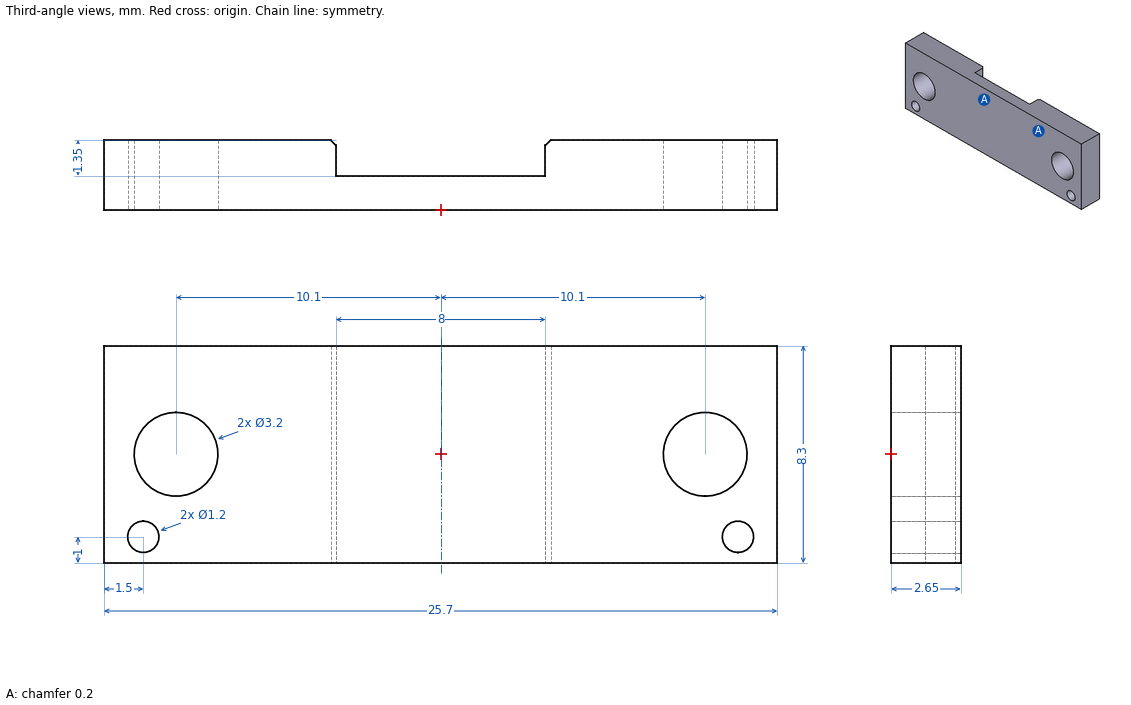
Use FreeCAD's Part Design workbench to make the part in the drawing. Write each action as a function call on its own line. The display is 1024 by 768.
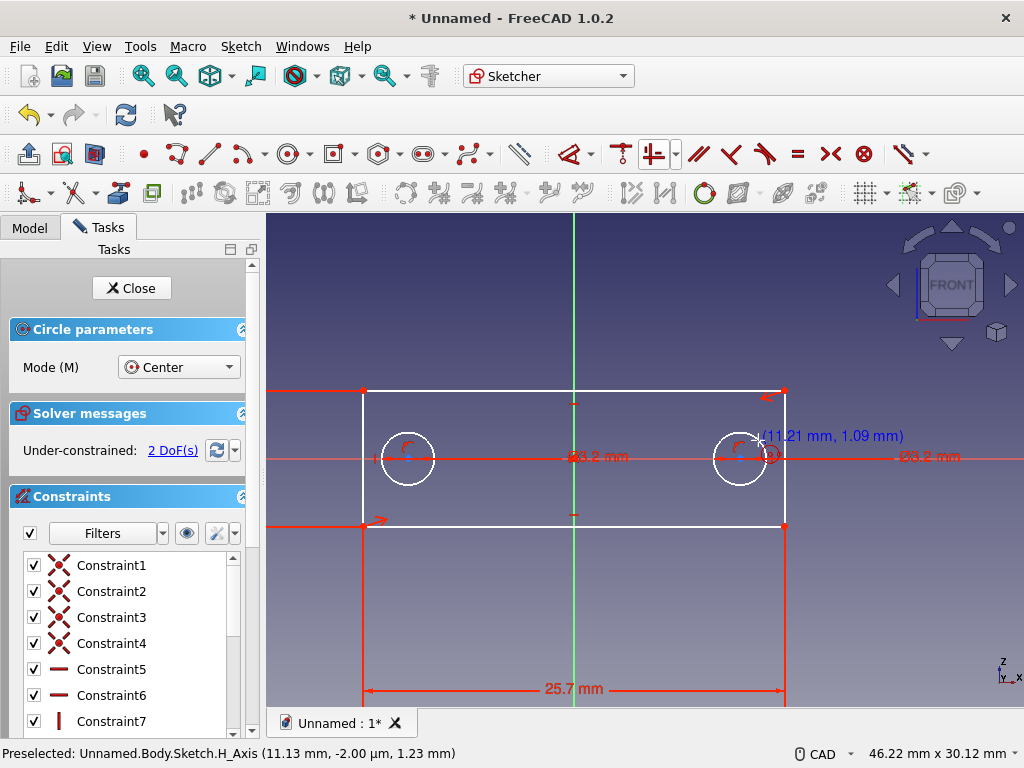
scroll(388, 511, up, 5)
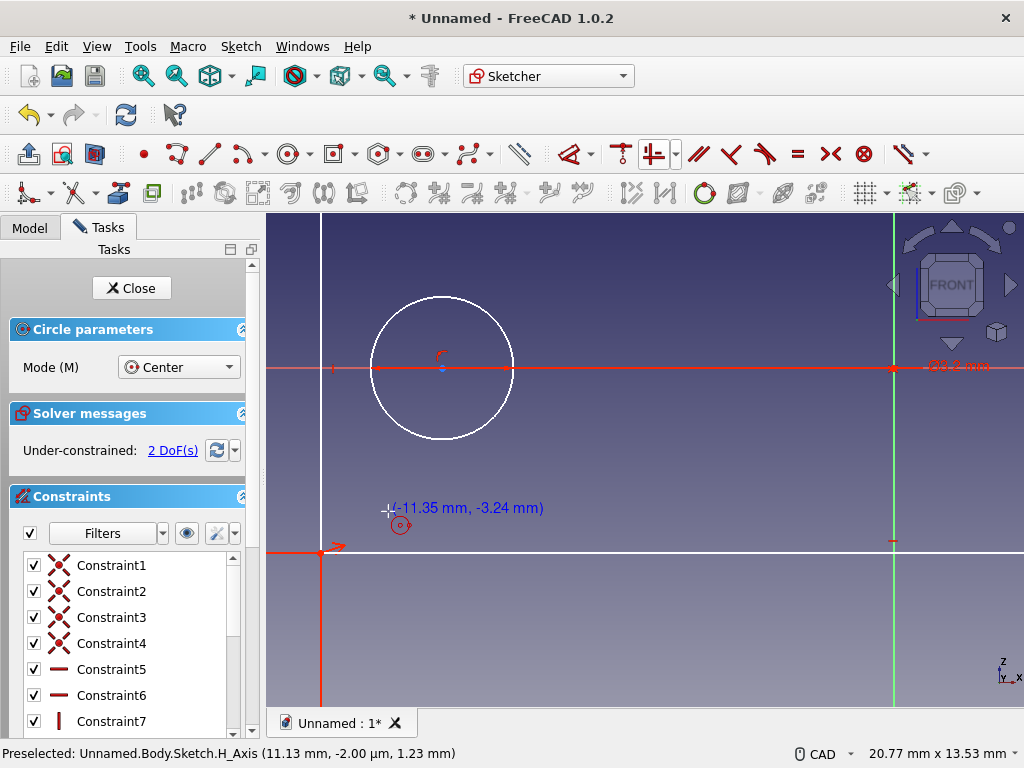
click(388, 509)
move(407, 490)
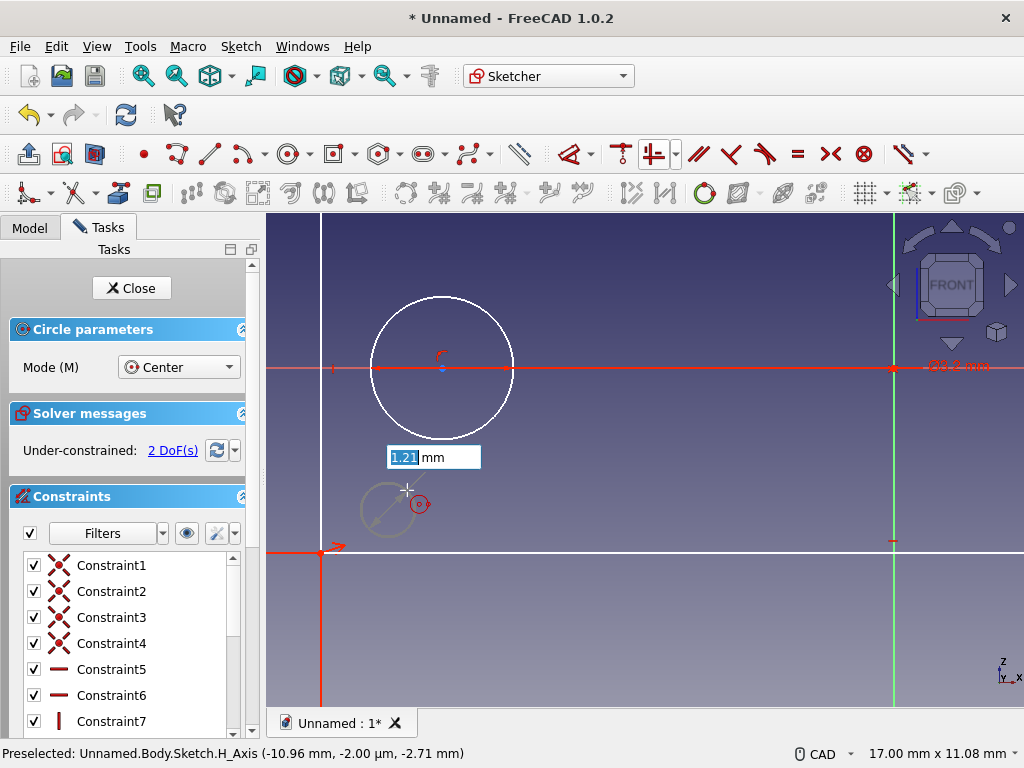
text(1.2)
key(Return)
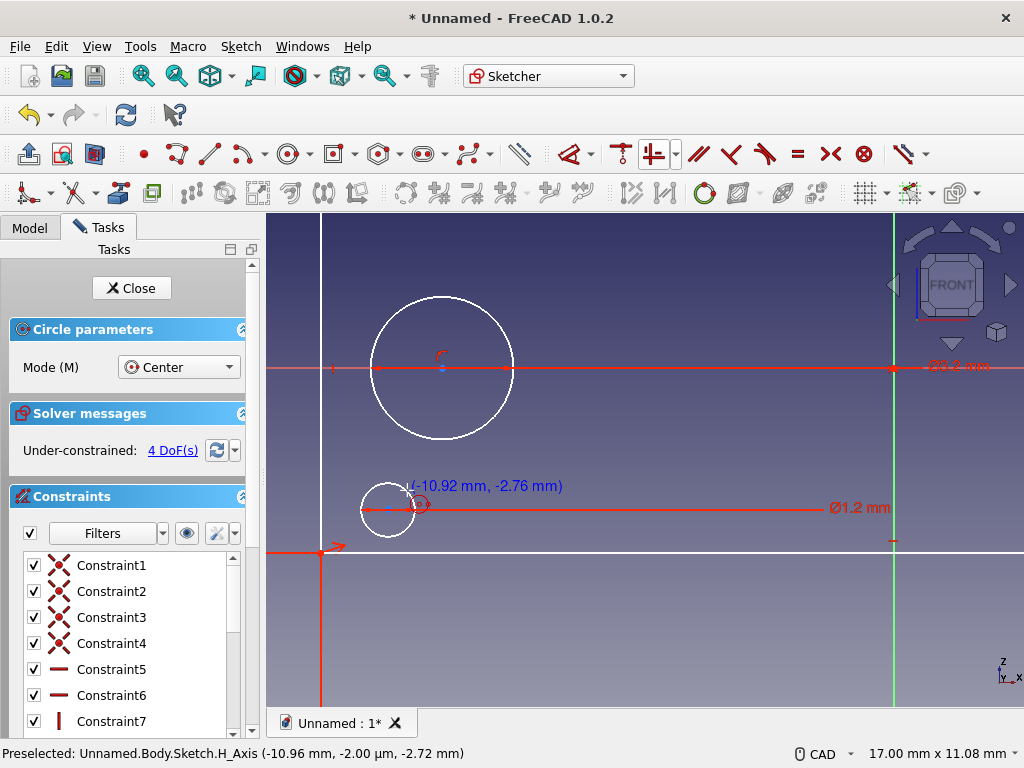
scroll(392, 513, down, 5)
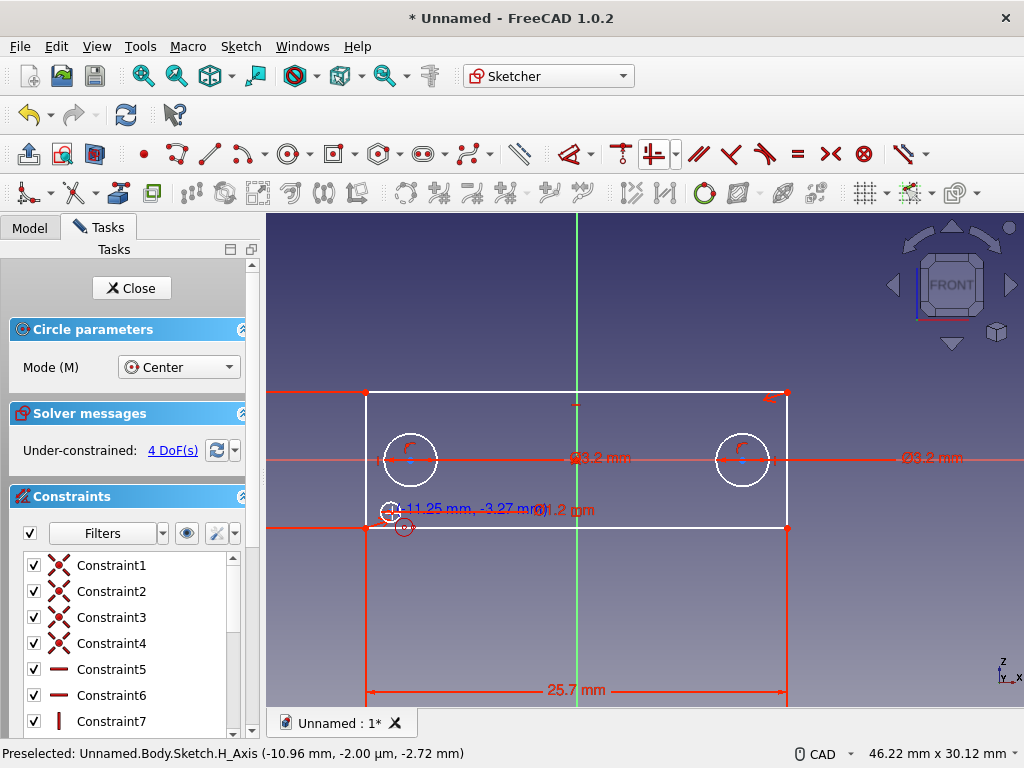
scroll(763, 512, up, 5)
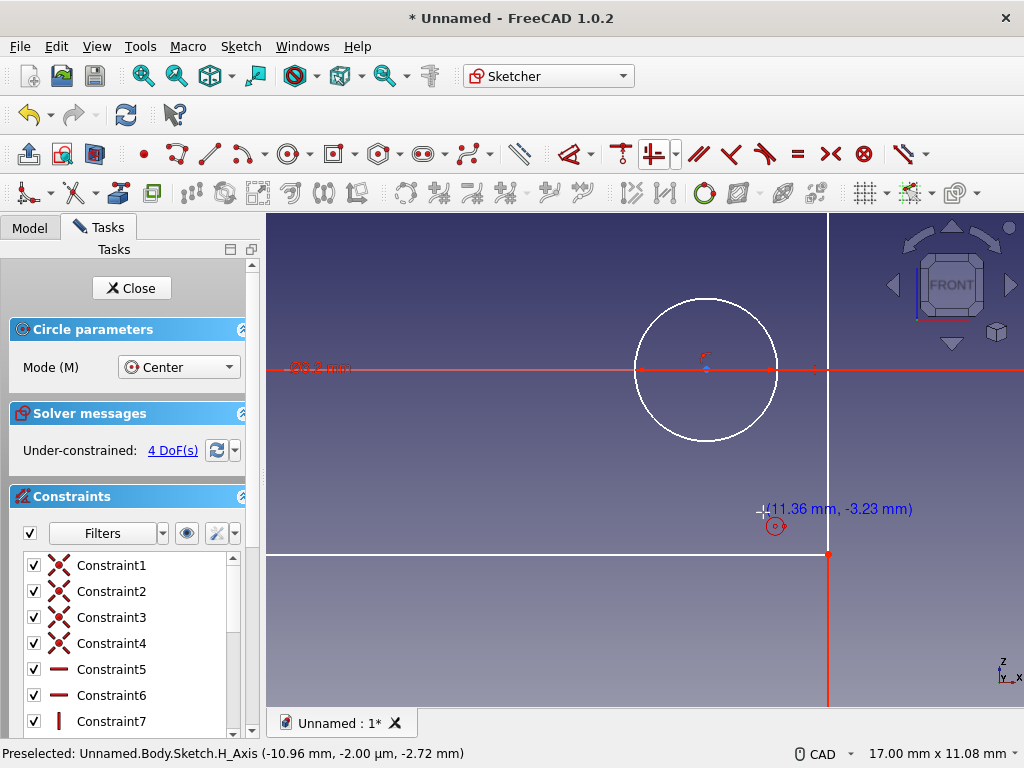
click(761, 510)
move(780, 491)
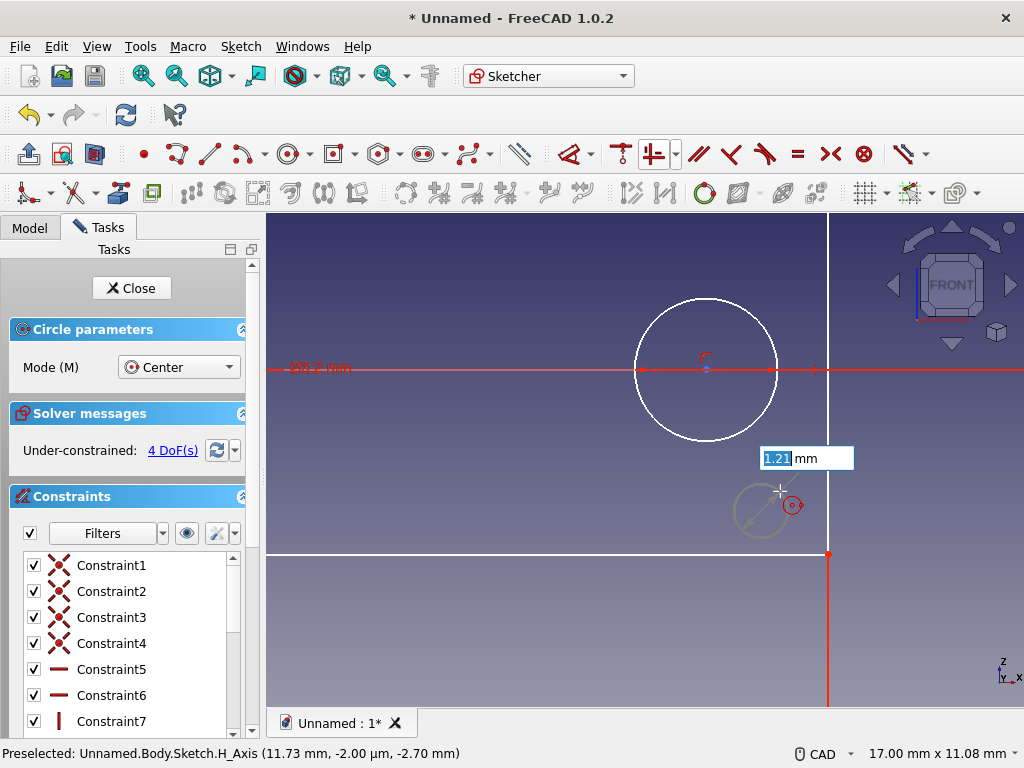
text(1.2)
key(Return)
key(Escape)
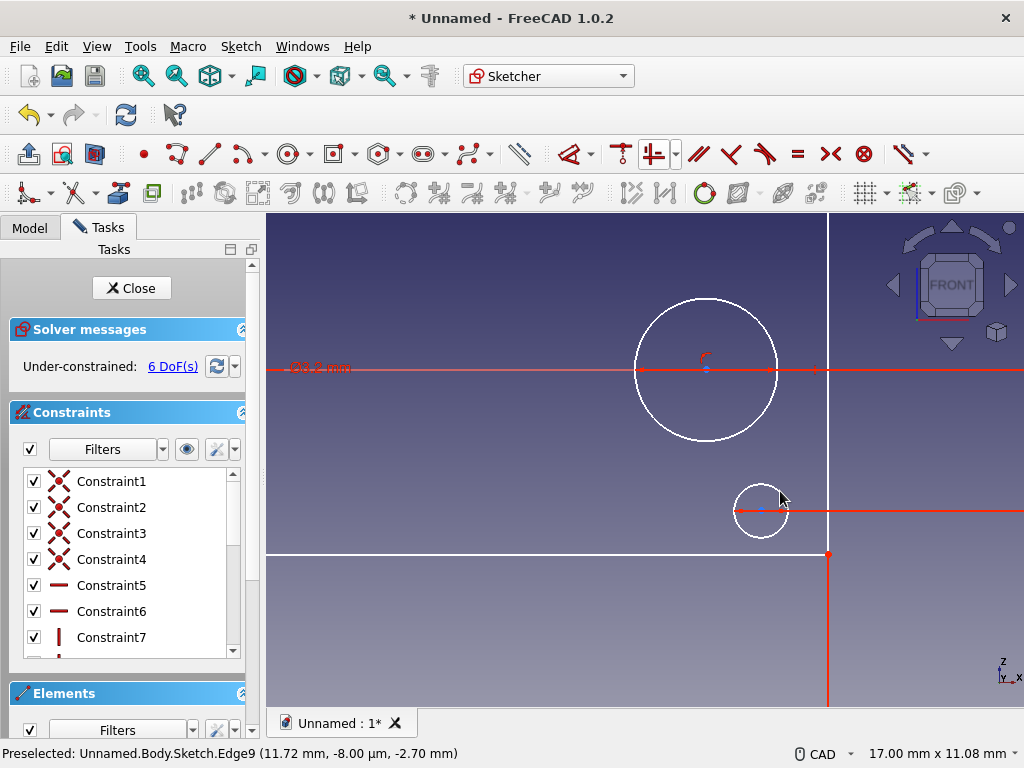
scroll(763, 512, down, 5)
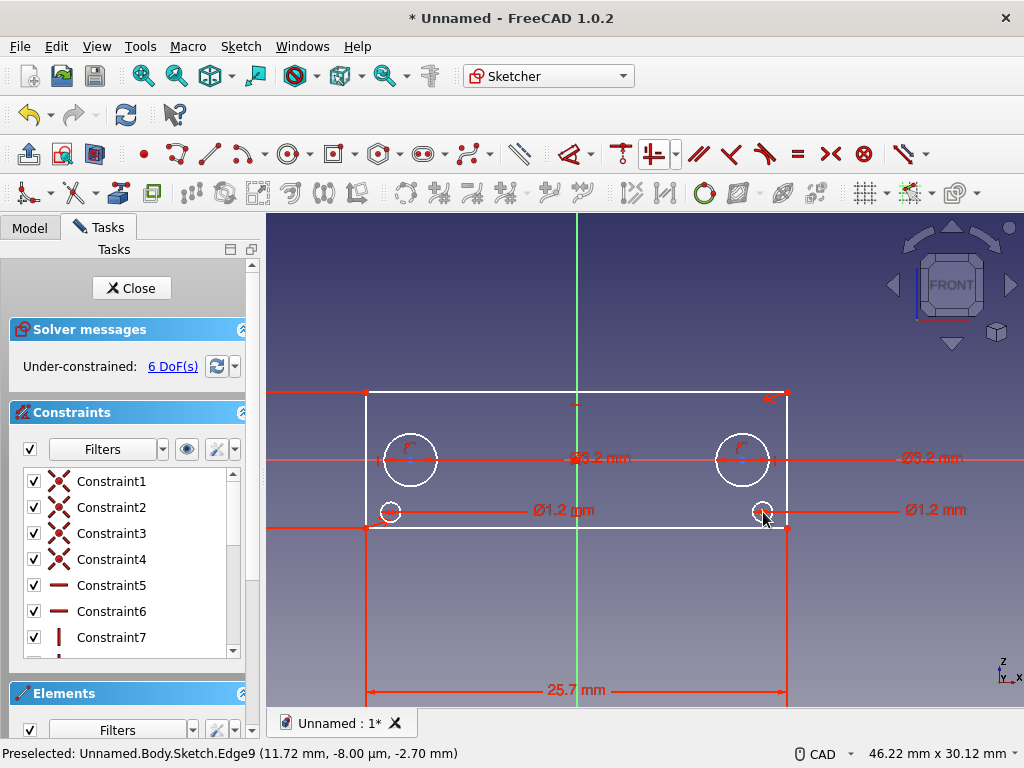
click(391, 512)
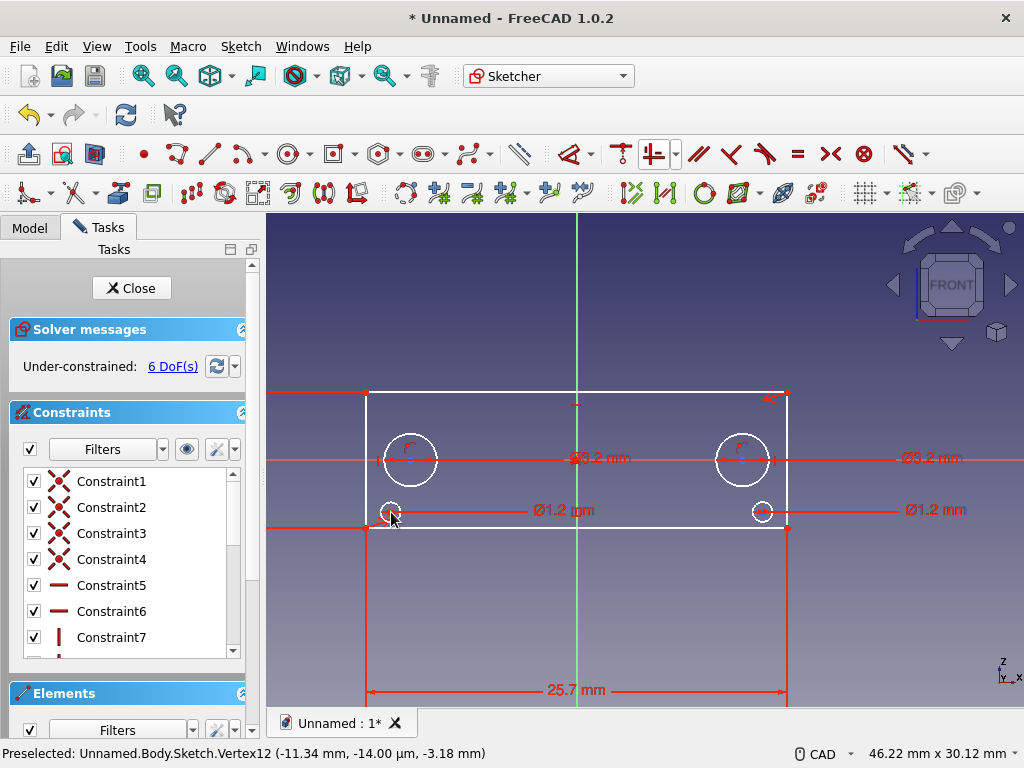
click(763, 512)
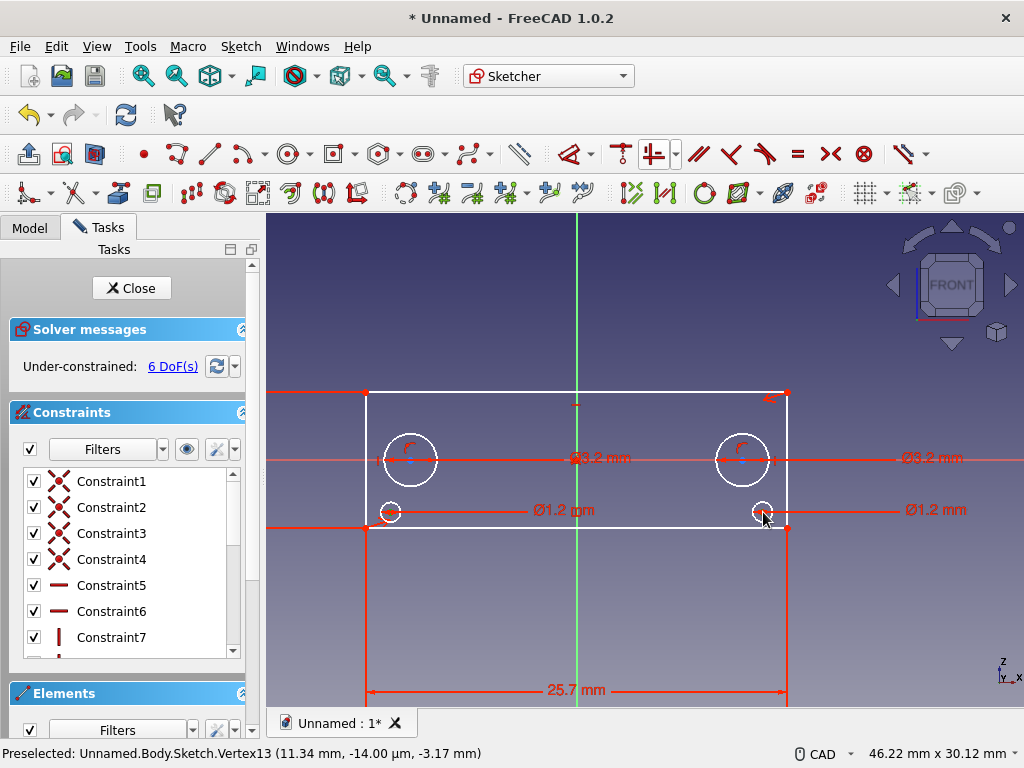
click(577, 648)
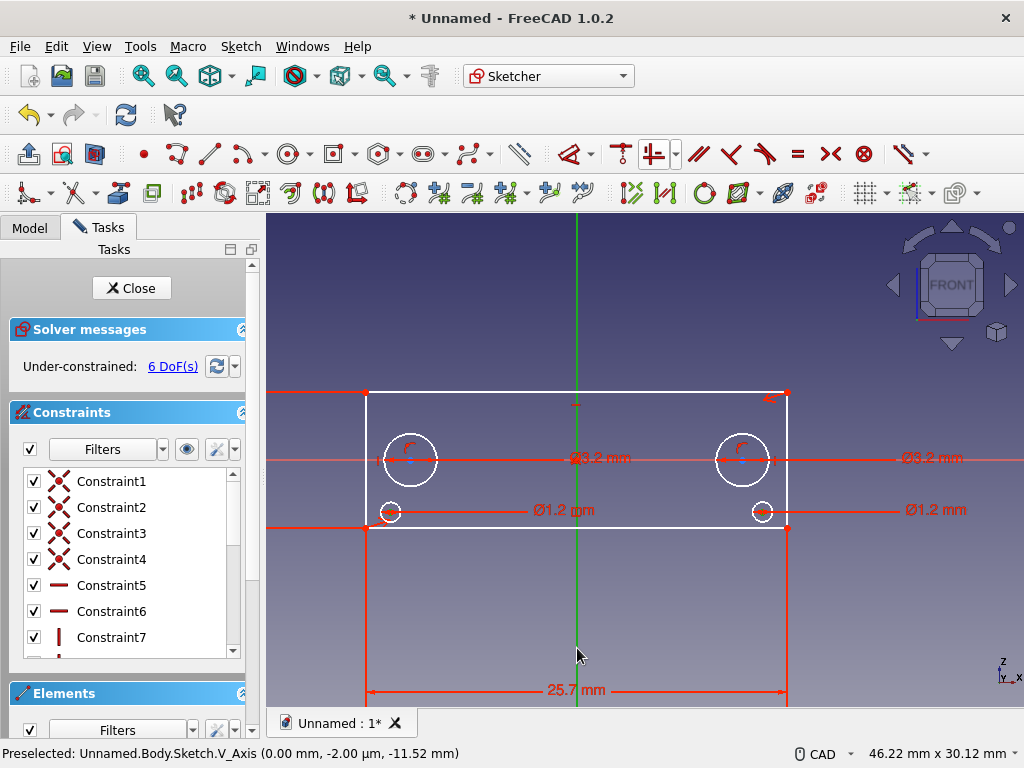
click(831, 154)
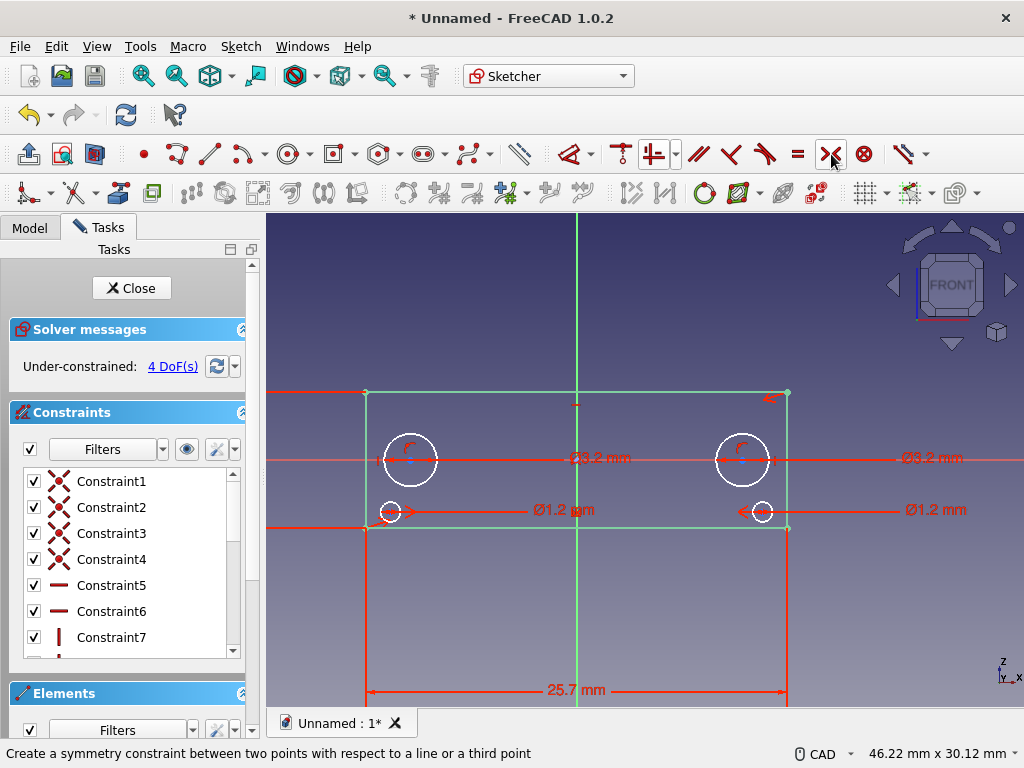
click(568, 154)